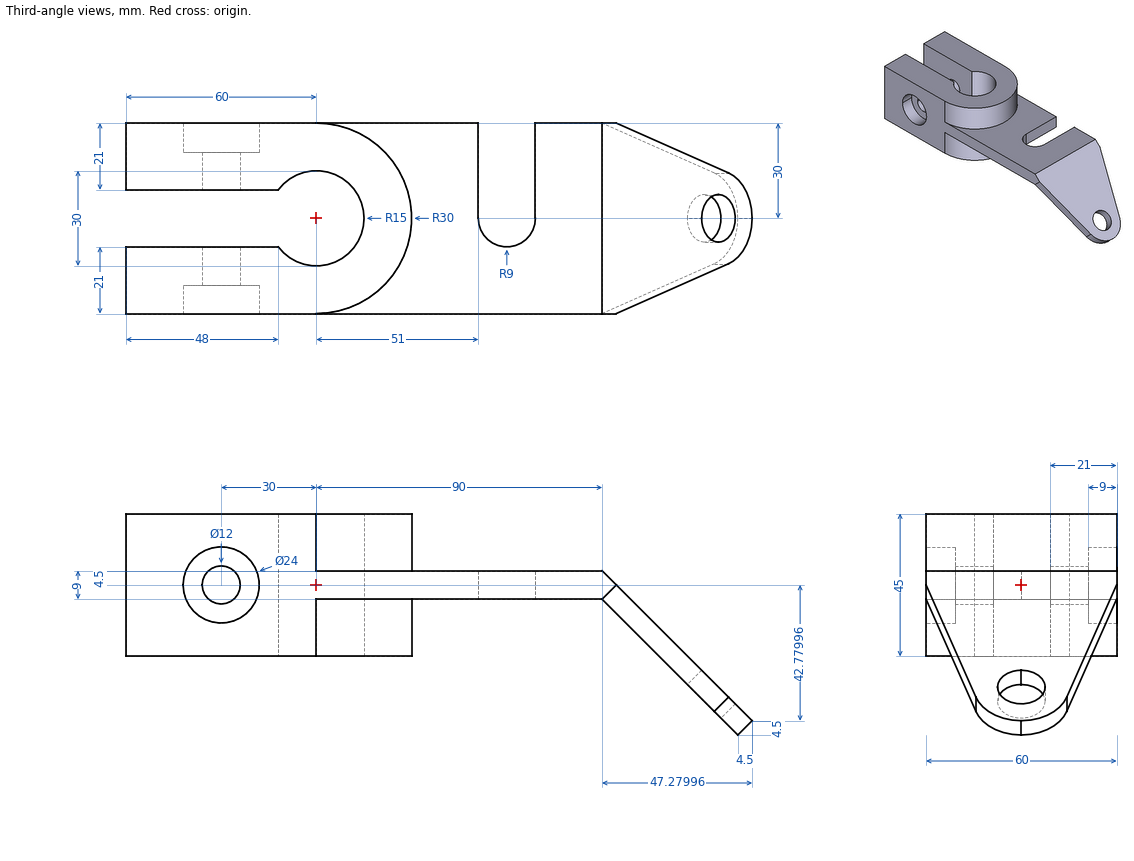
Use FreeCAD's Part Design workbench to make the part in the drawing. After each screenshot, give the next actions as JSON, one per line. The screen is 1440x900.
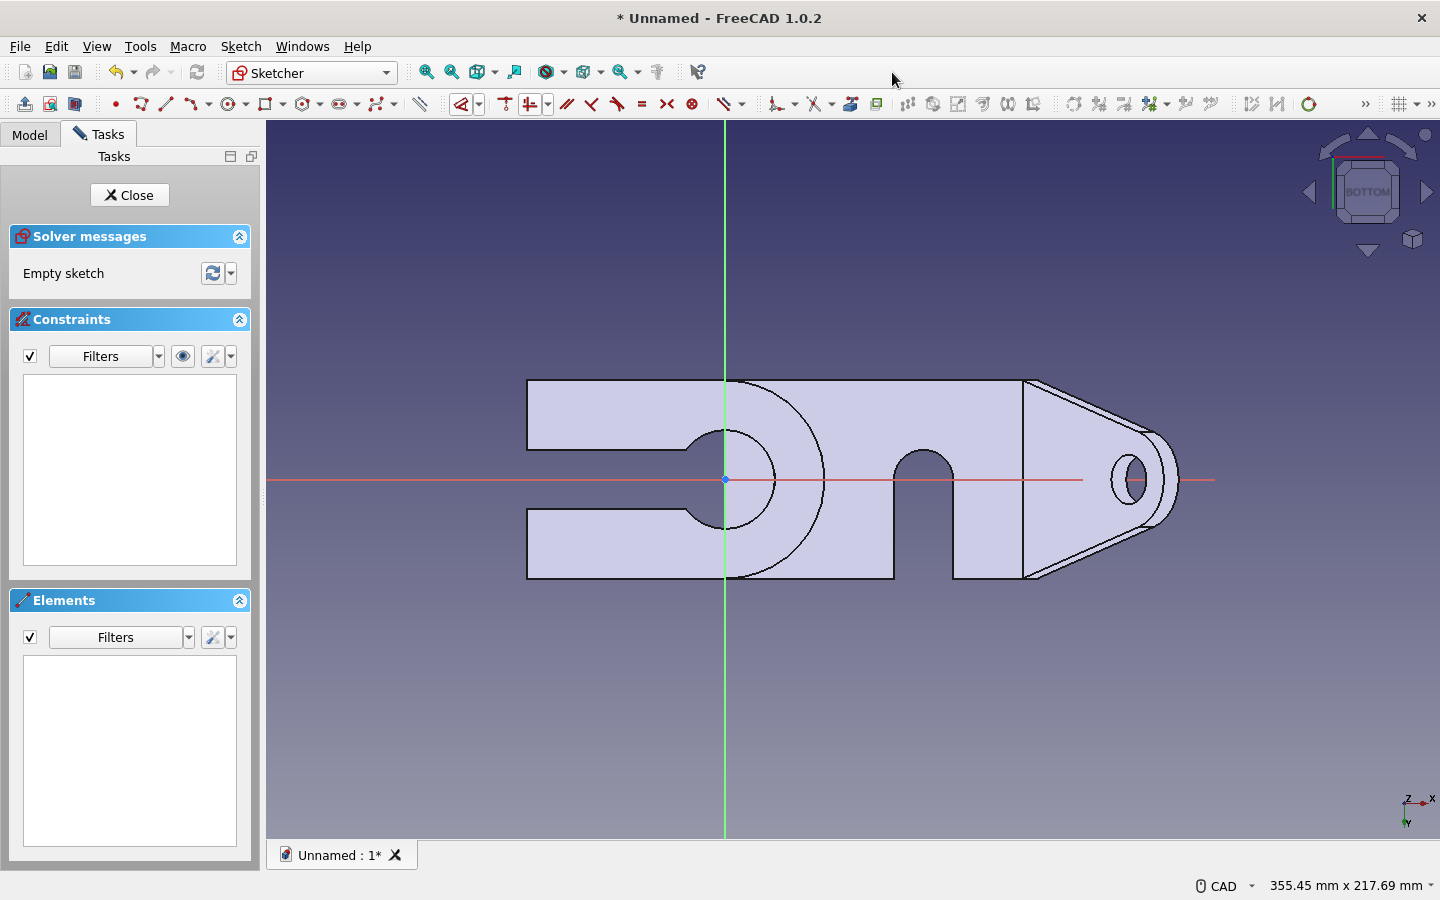
{"action": "left_click", "coordinate": [75, 104]}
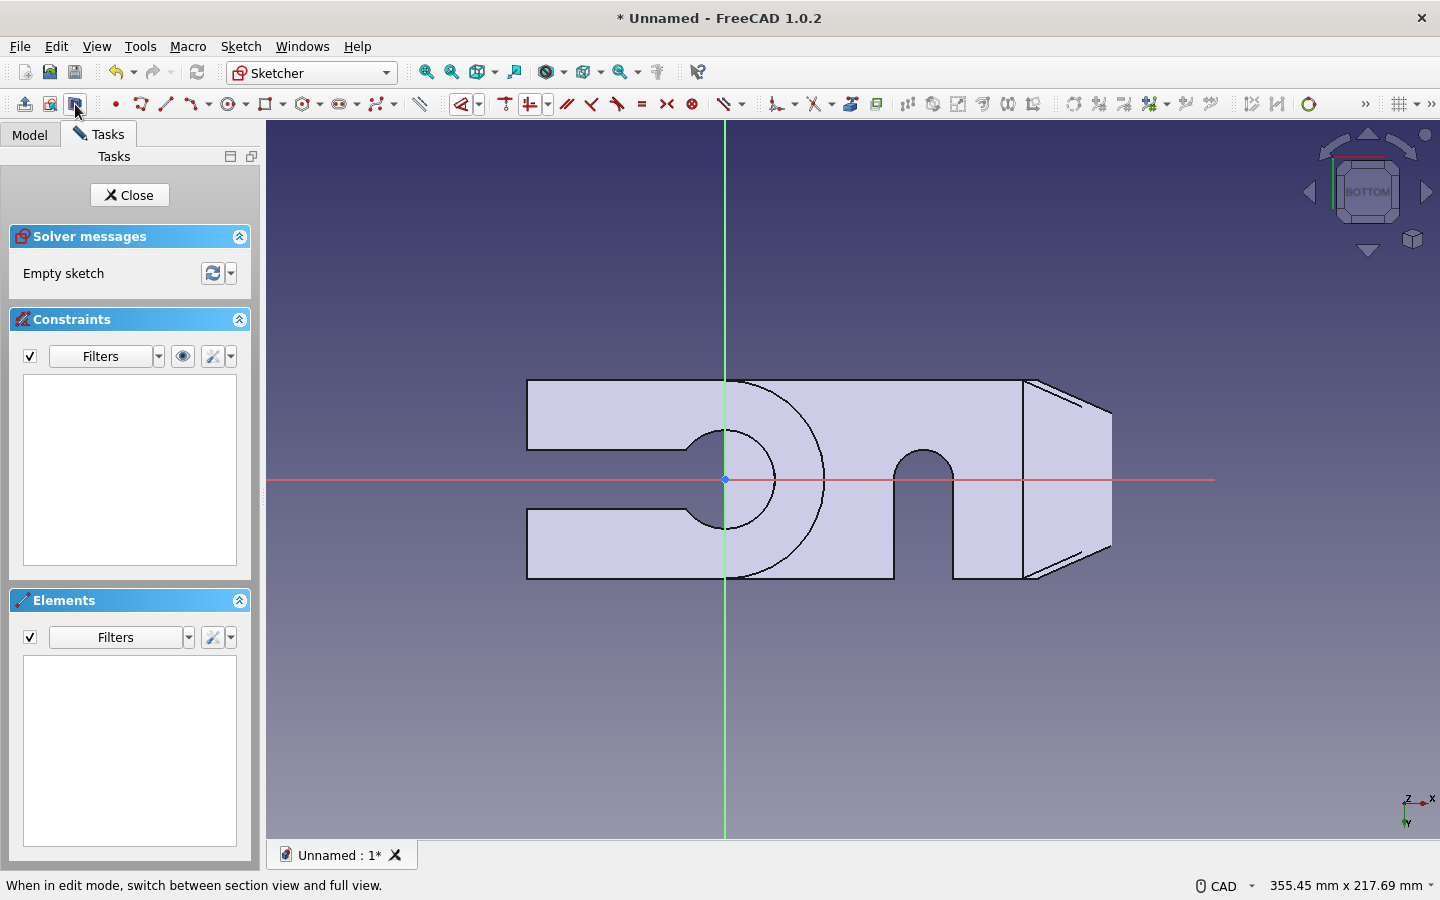
{"action": "scroll", "coordinate": [741, 480], "scroll_direction": "up", "scroll_amount": 8}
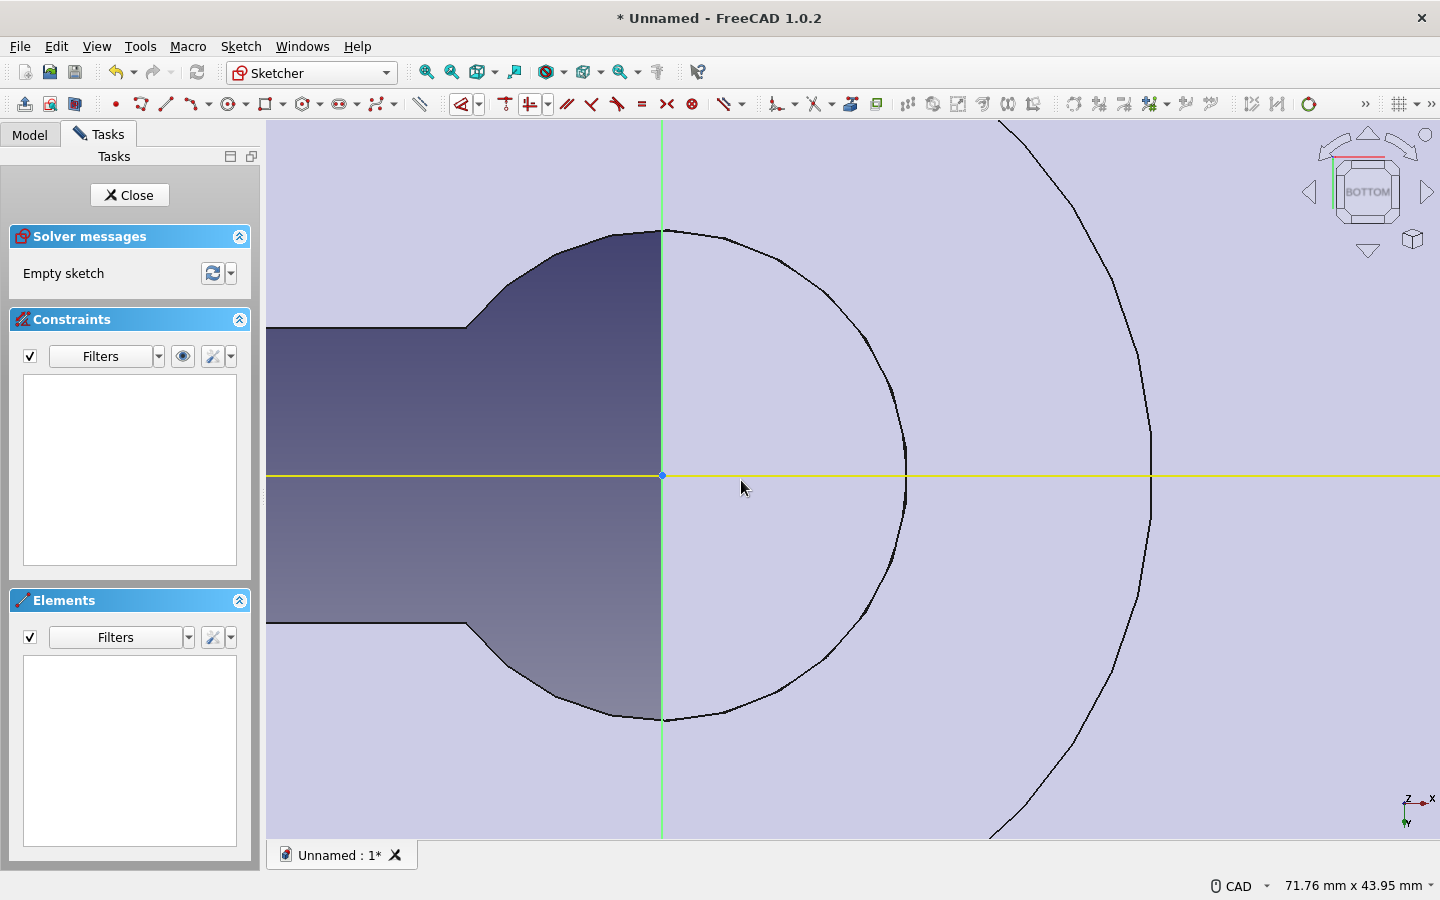
{"action": "left_click", "coordinate": [166, 104]}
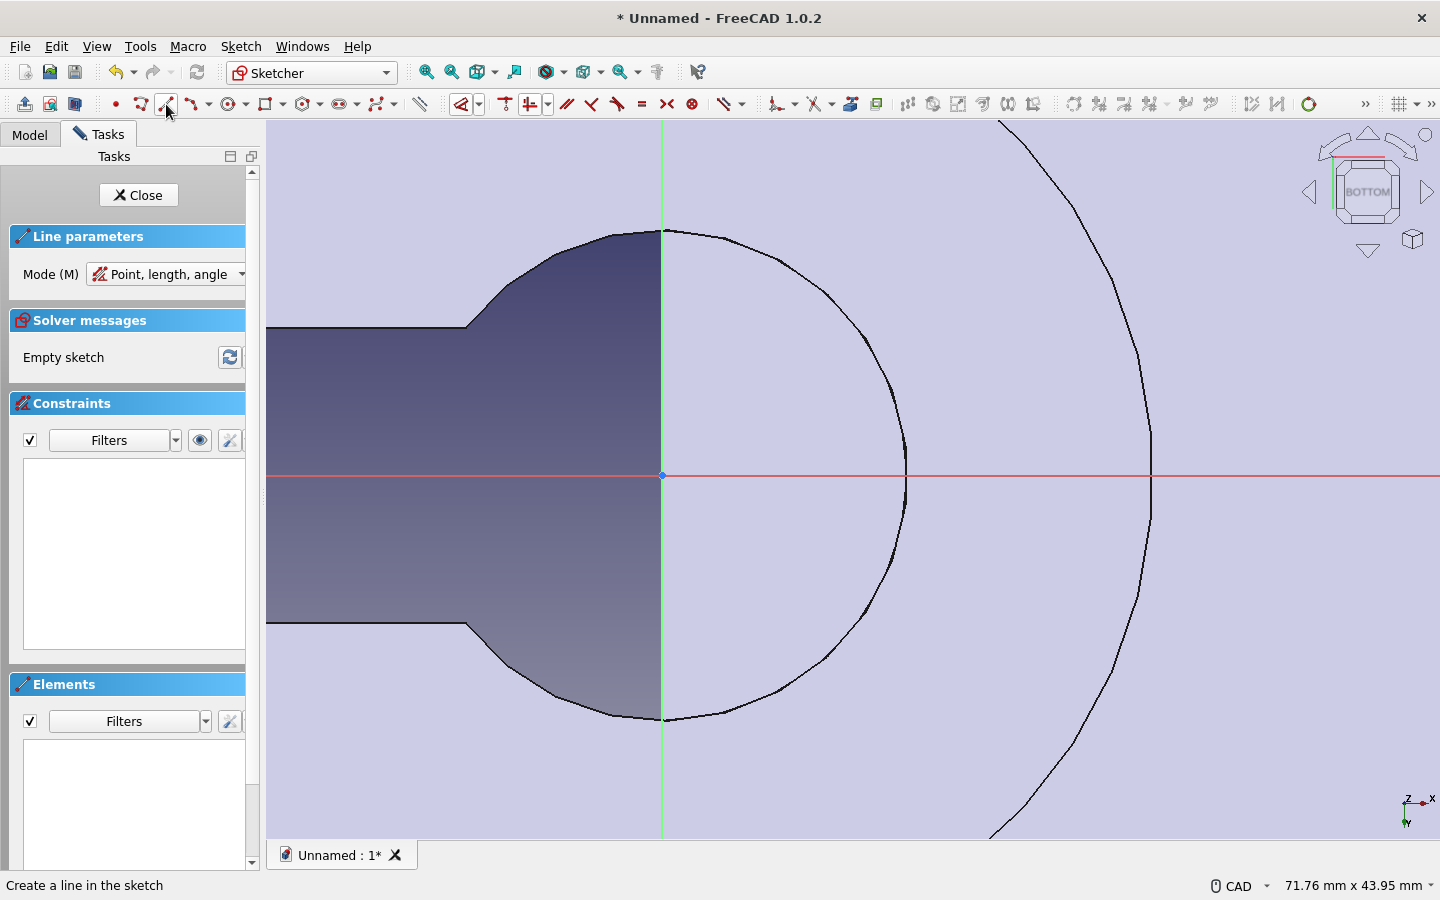
{"action": "left_click", "coordinate": [662, 230]}
{"action": "left_click", "coordinate": [671, 721]}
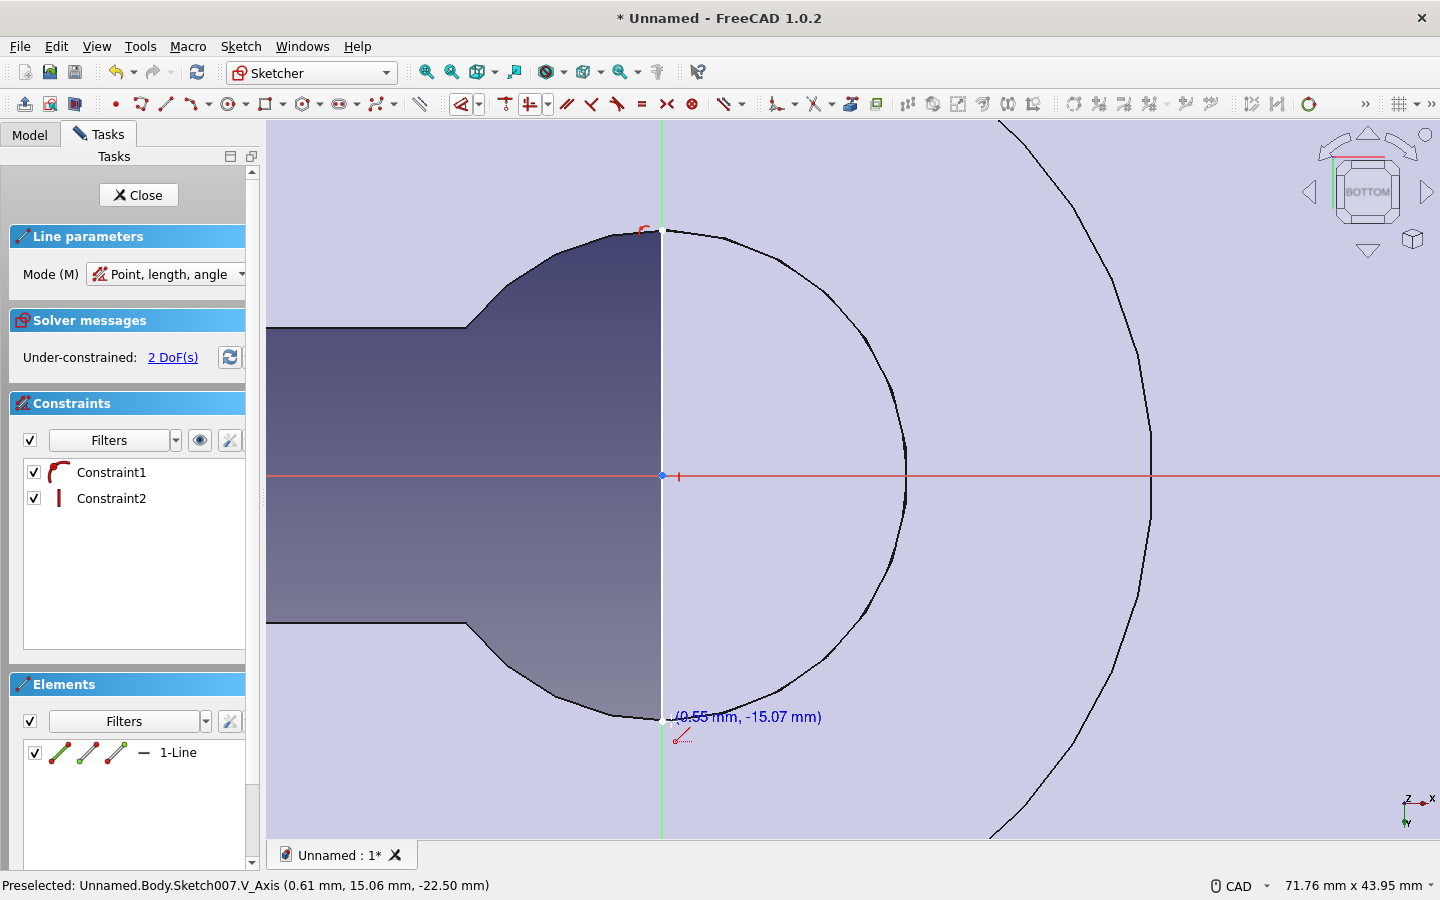
{"action": "left_click", "coordinate": [190, 104]}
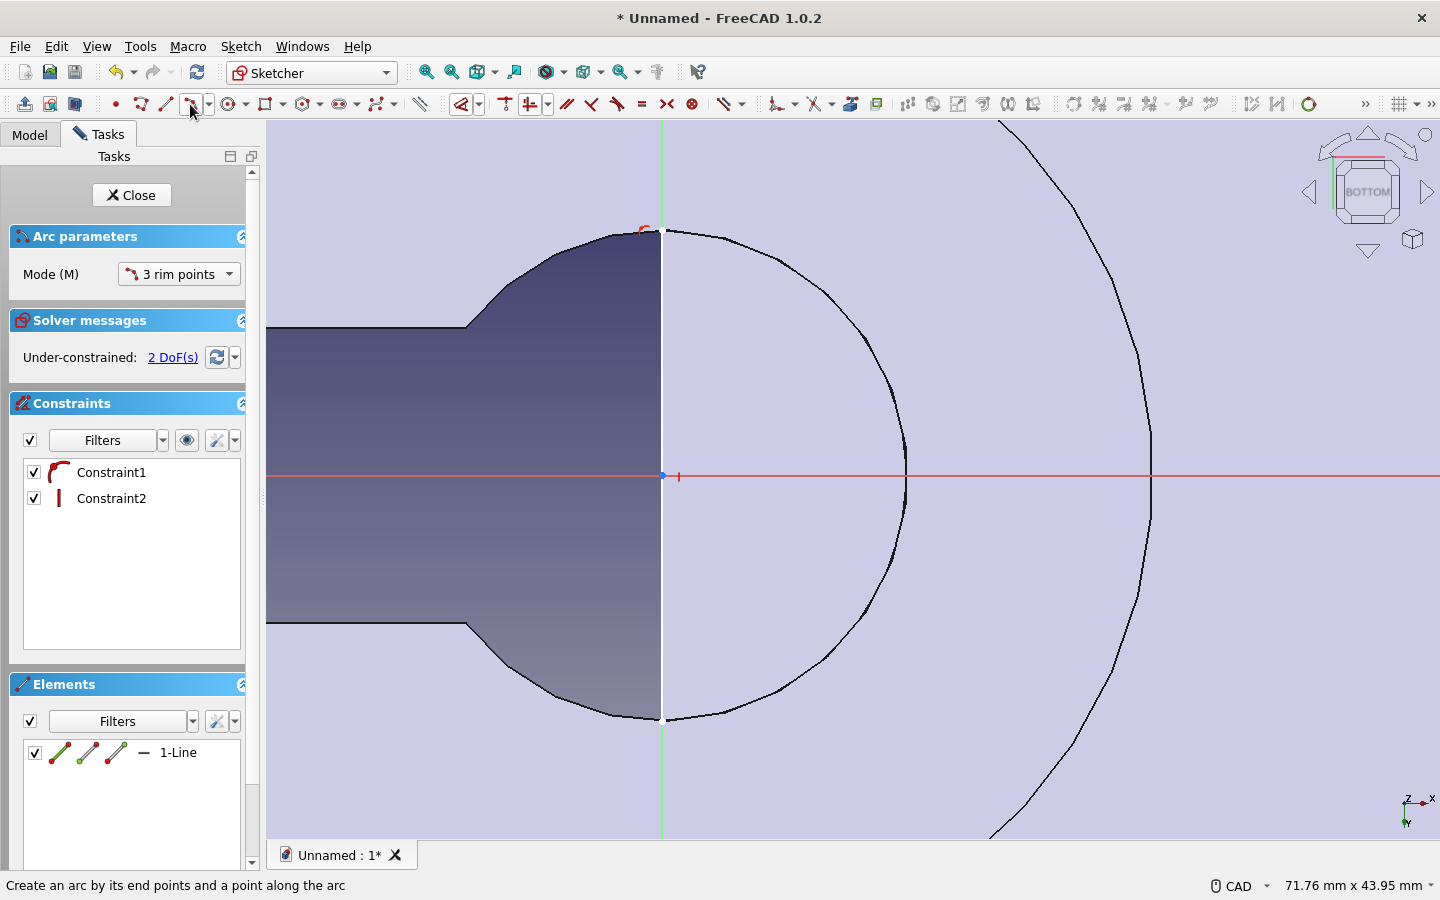
{"action": "left_click", "coordinate": [671, 721]}
{"action": "left_click", "coordinate": [662, 231]}
{"action": "left_click", "coordinate": [895, 551]}
{"action": "key", "text": "Escape"}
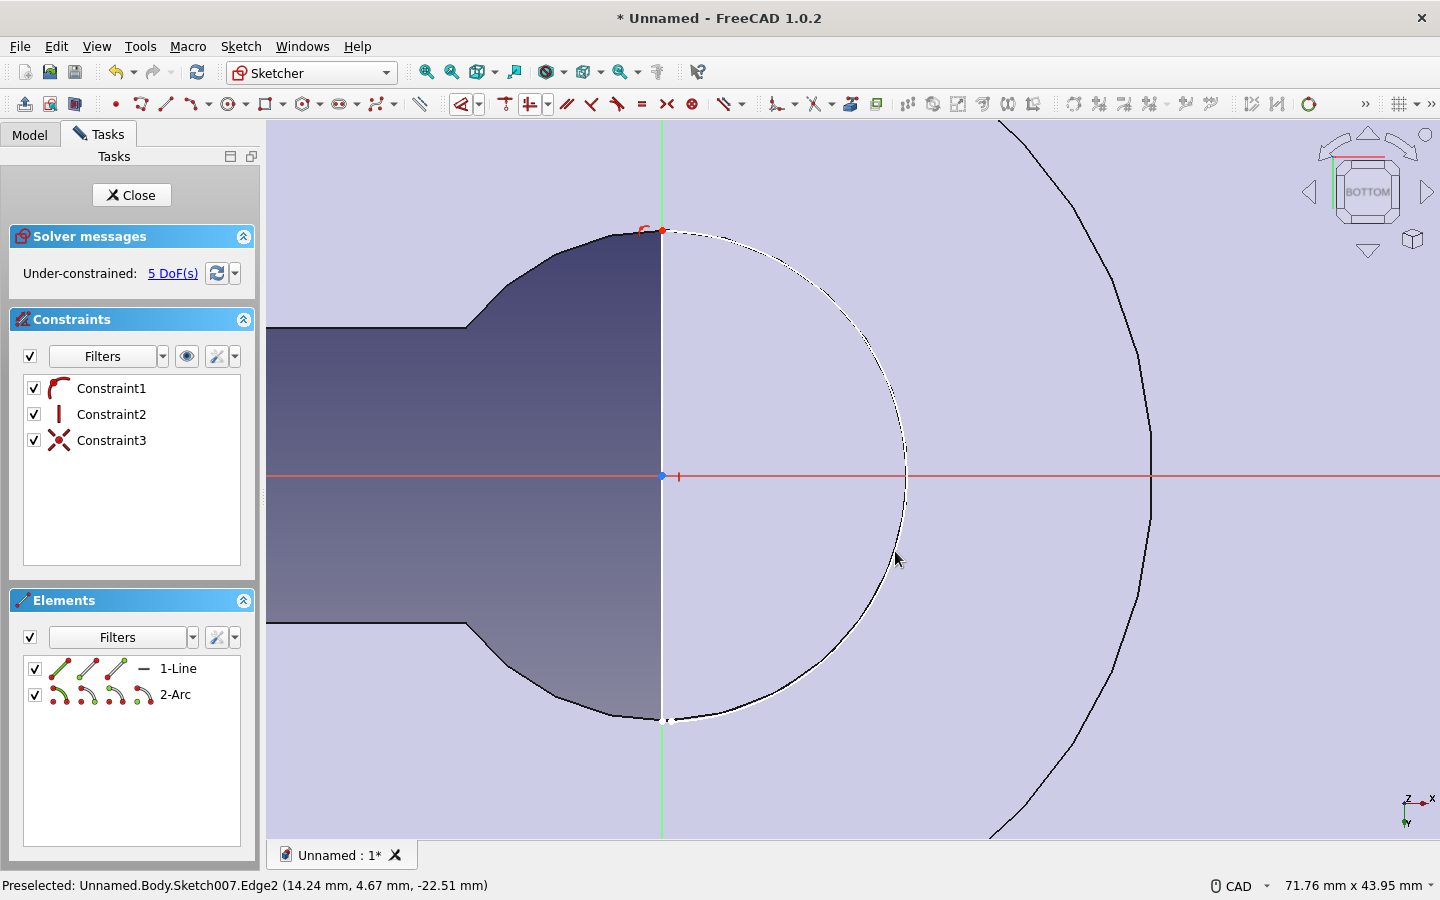
{"action": "left_click_drag", "start_coordinate": [651, 466], "coordinate": [672, 487]}